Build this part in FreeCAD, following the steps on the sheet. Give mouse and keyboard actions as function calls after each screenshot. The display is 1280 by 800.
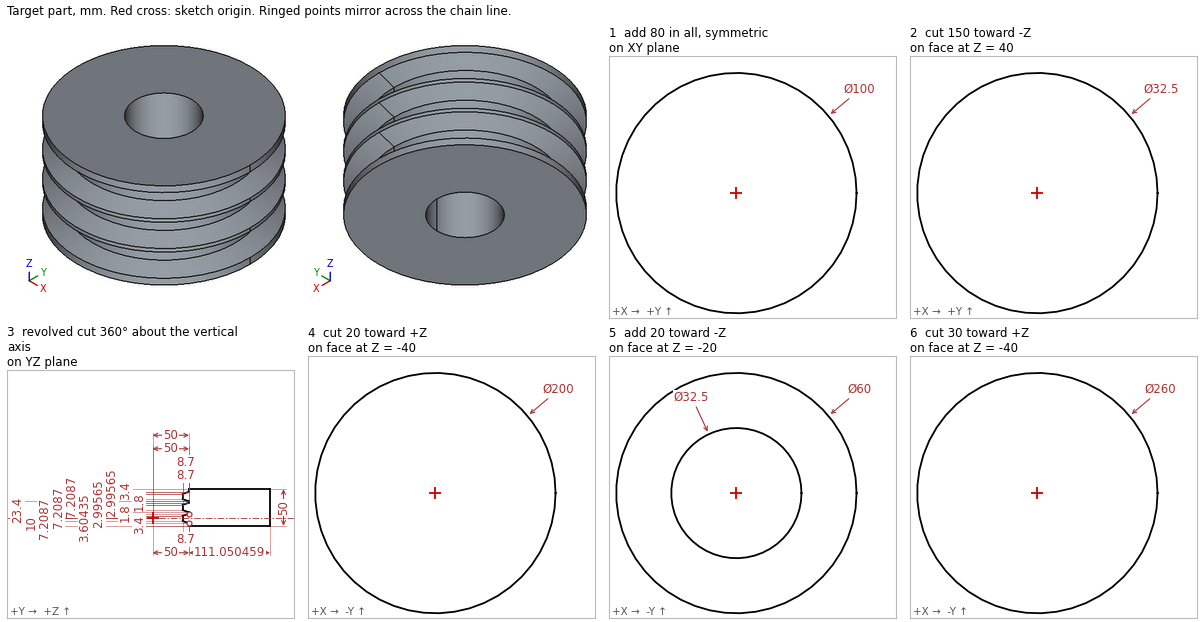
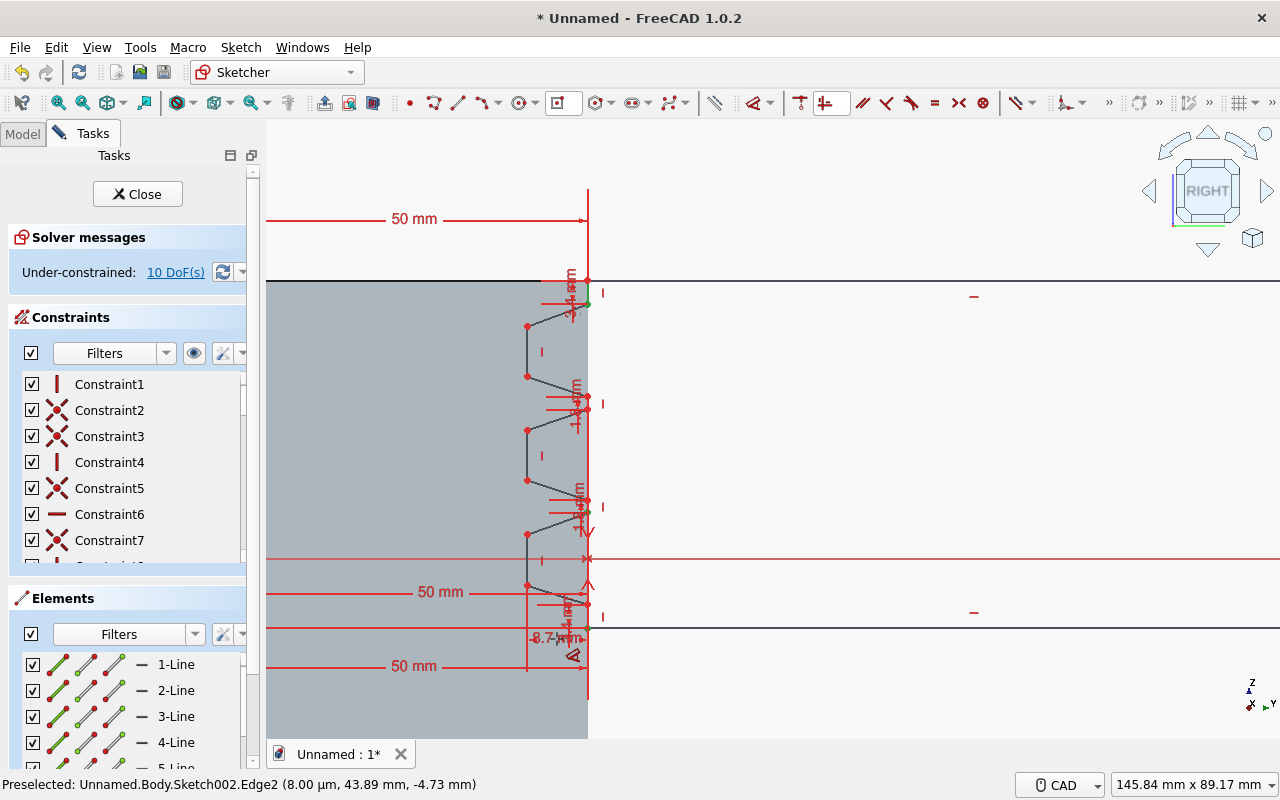
click(570, 311)
click(557, 270)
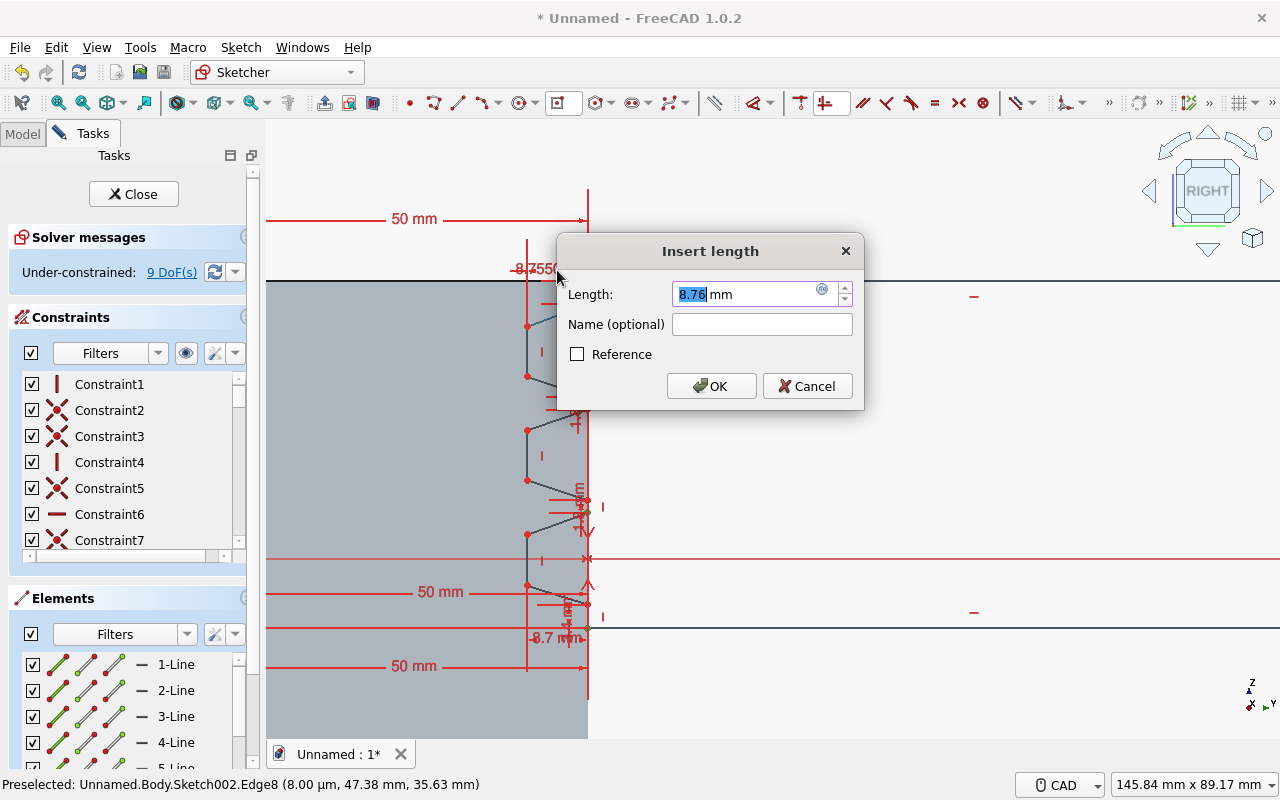
text(8.7)
key(Return)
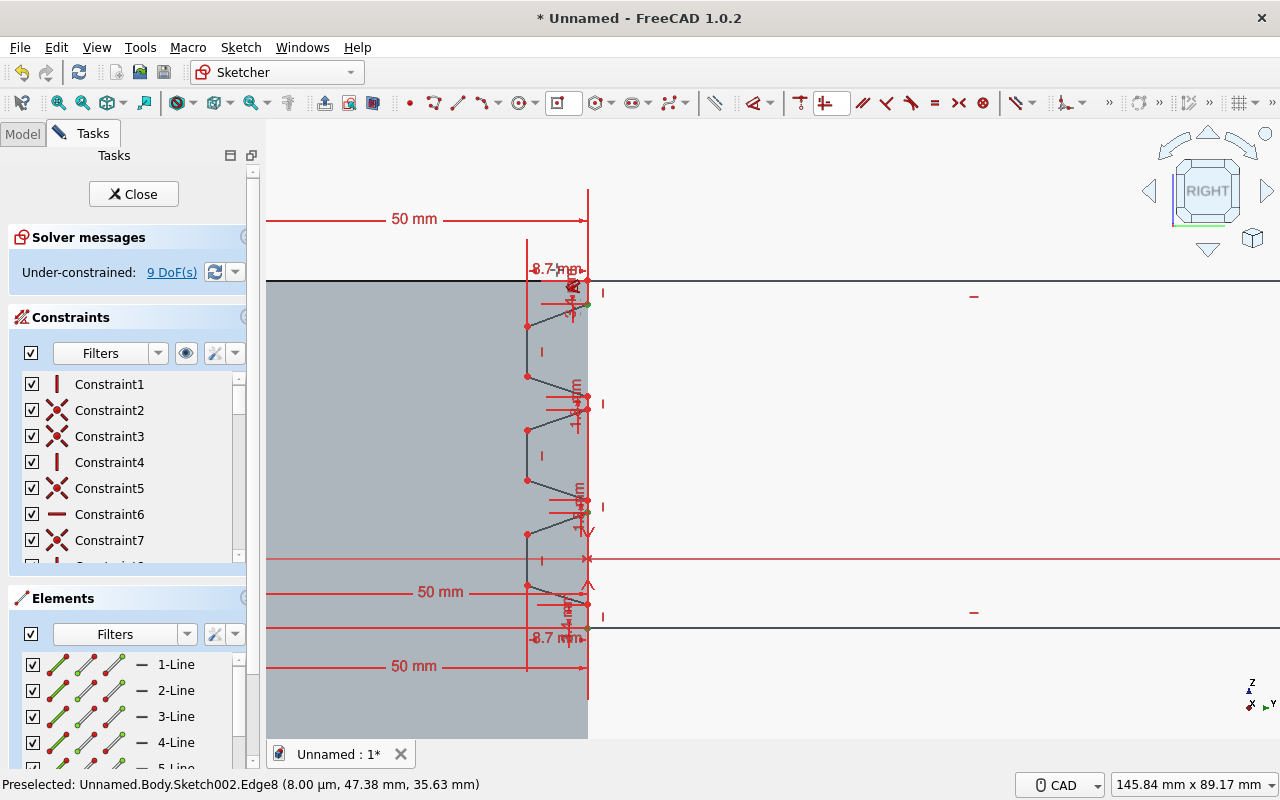
click(570, 416)
click(572, 376)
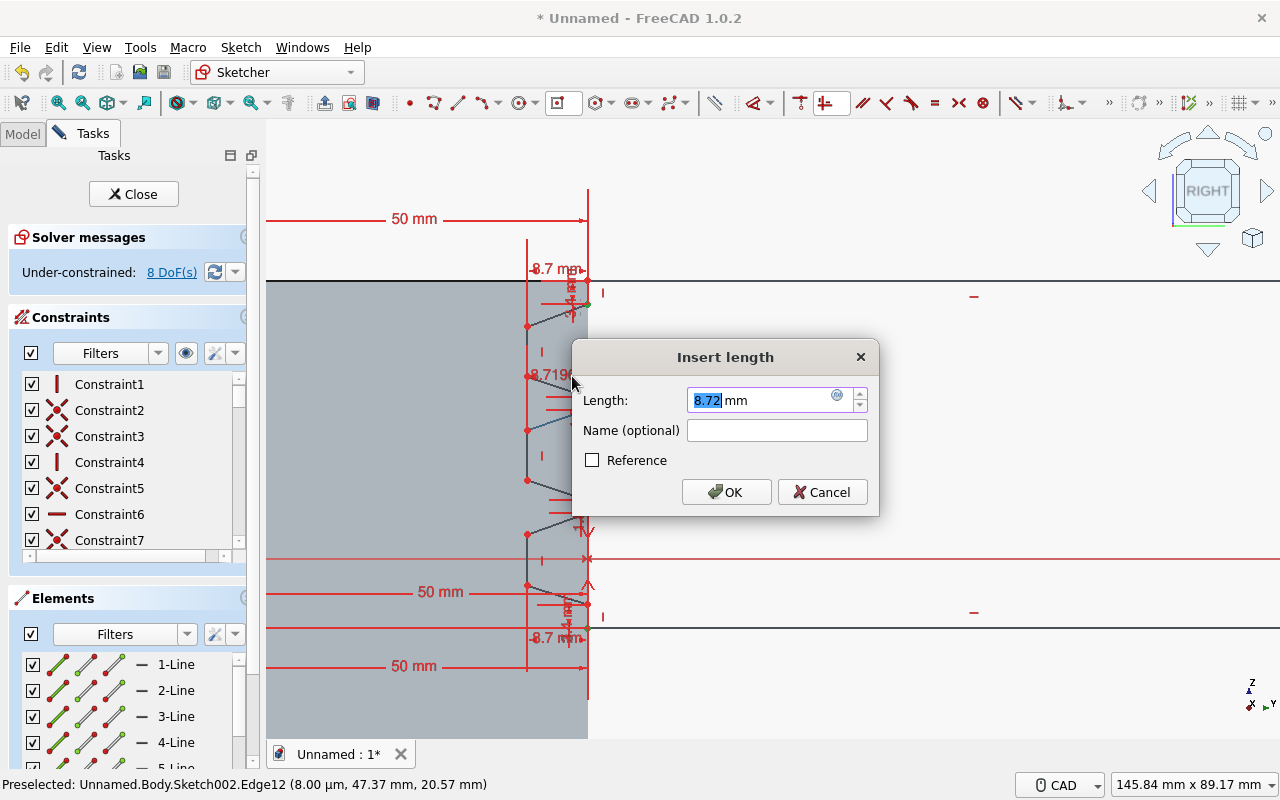
text(8.7)
key(Return)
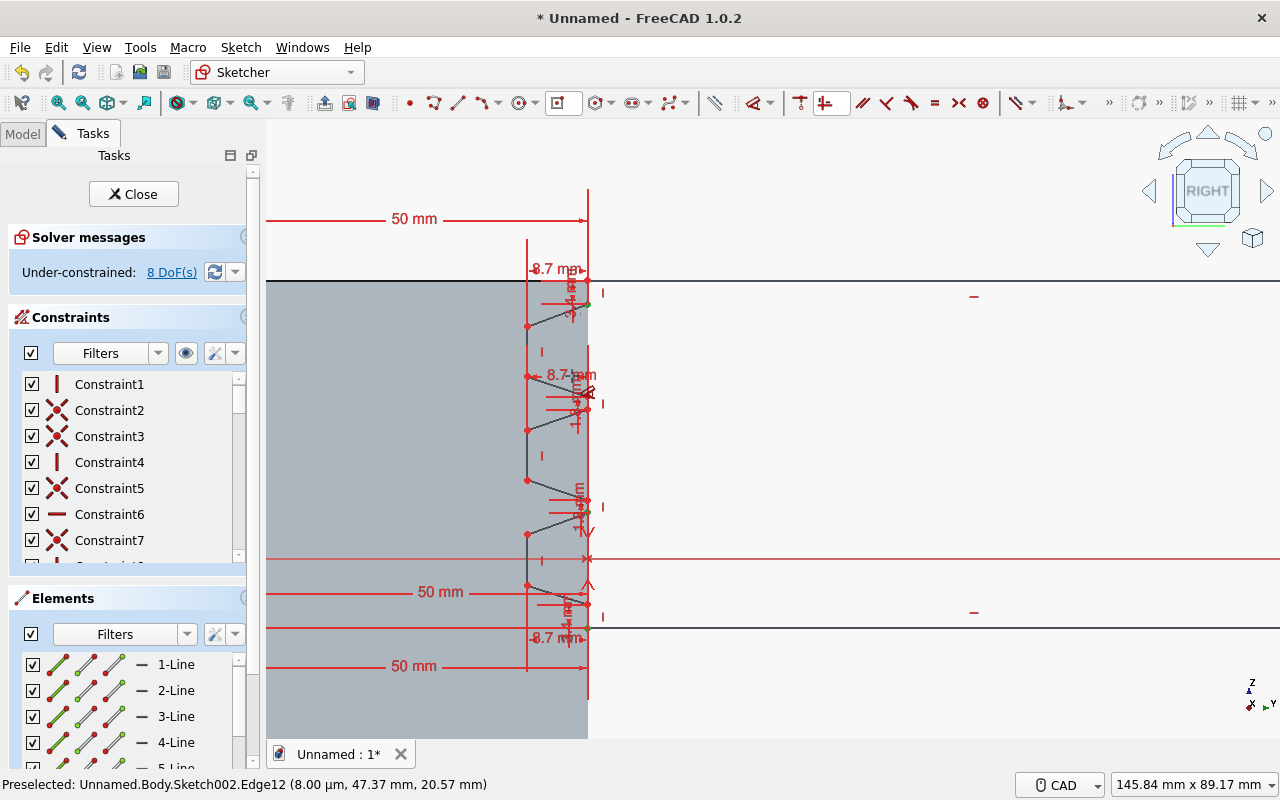
click(588, 397)
click(622, 478)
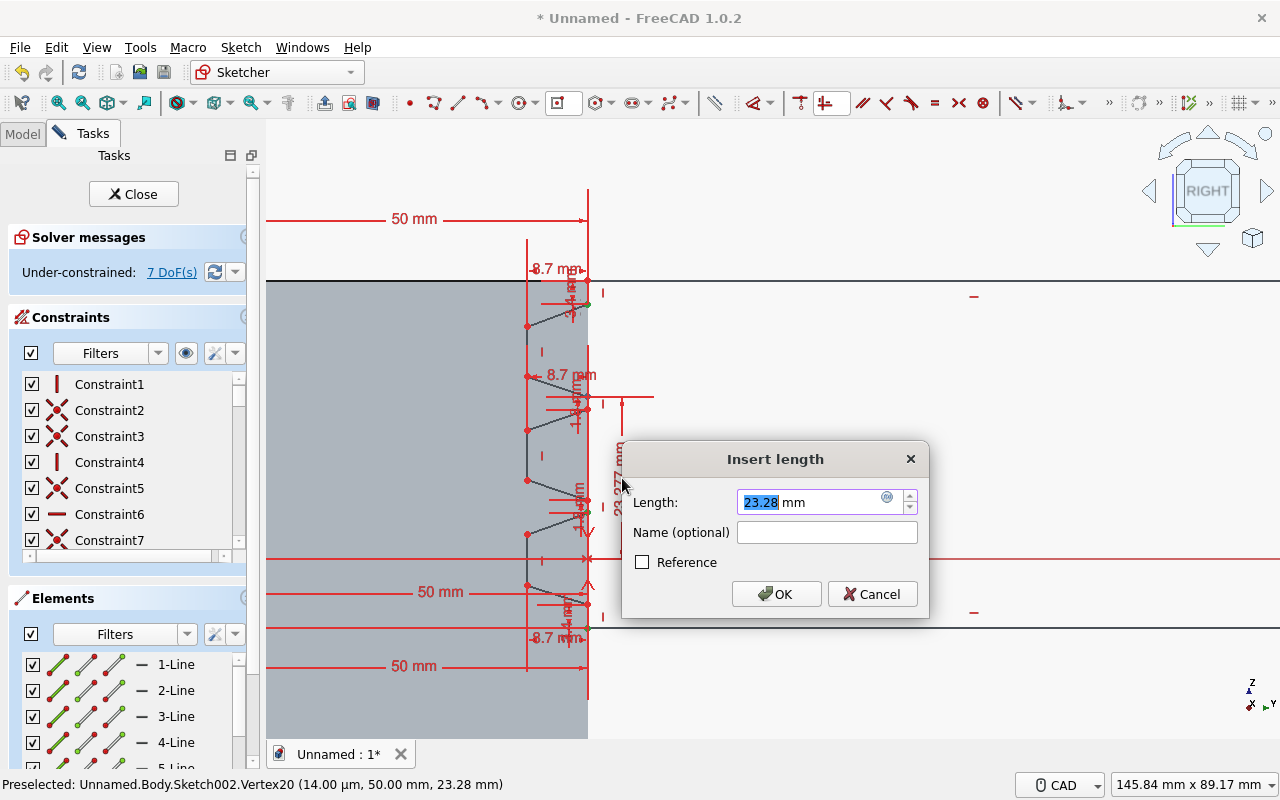
text(23.4)
key(Return)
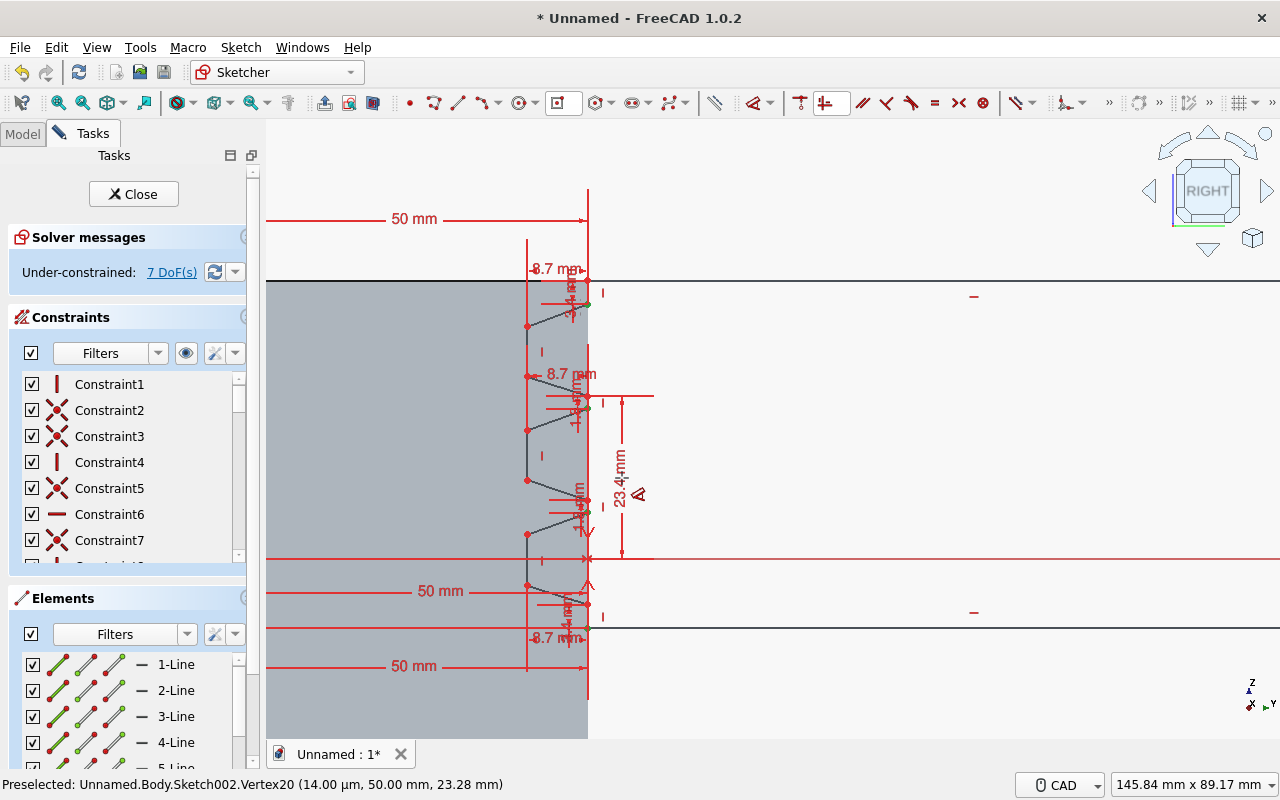
click(527, 571)
click(493, 572)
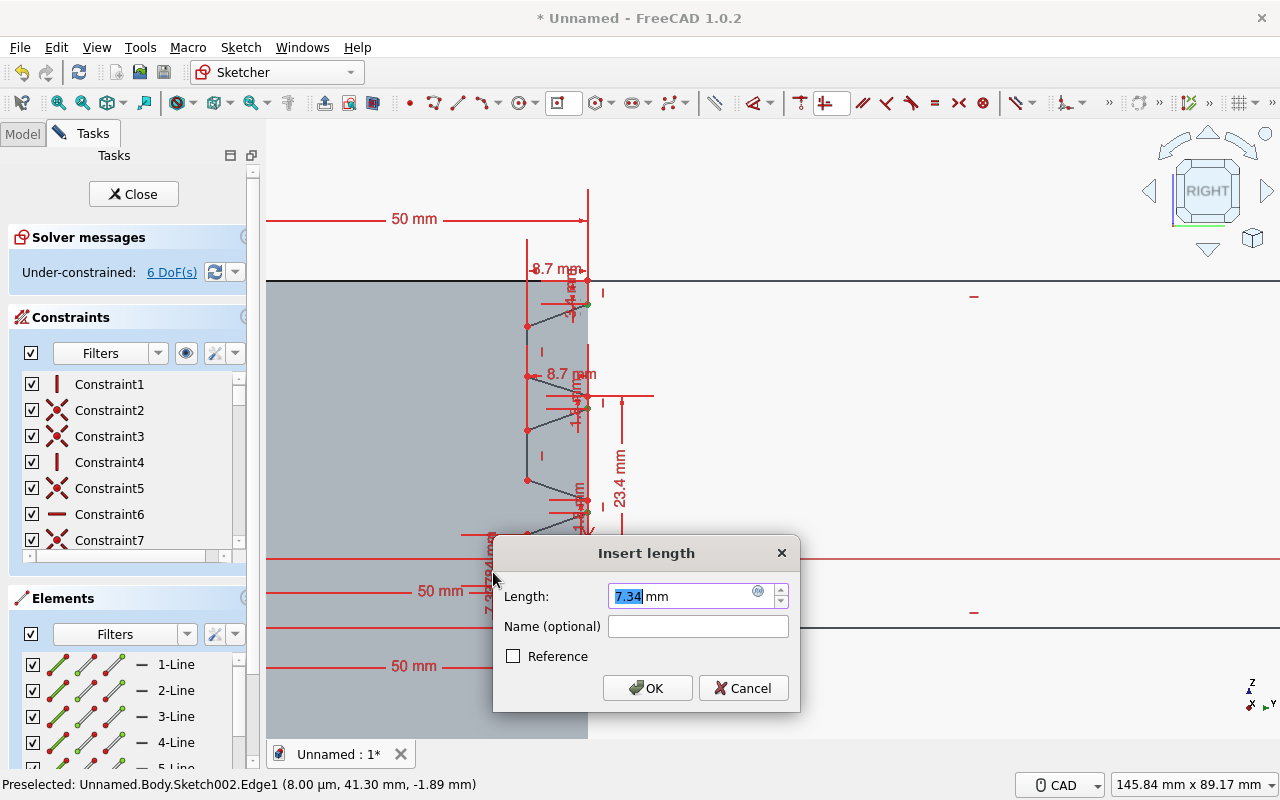
text(7.2087)
key(Return)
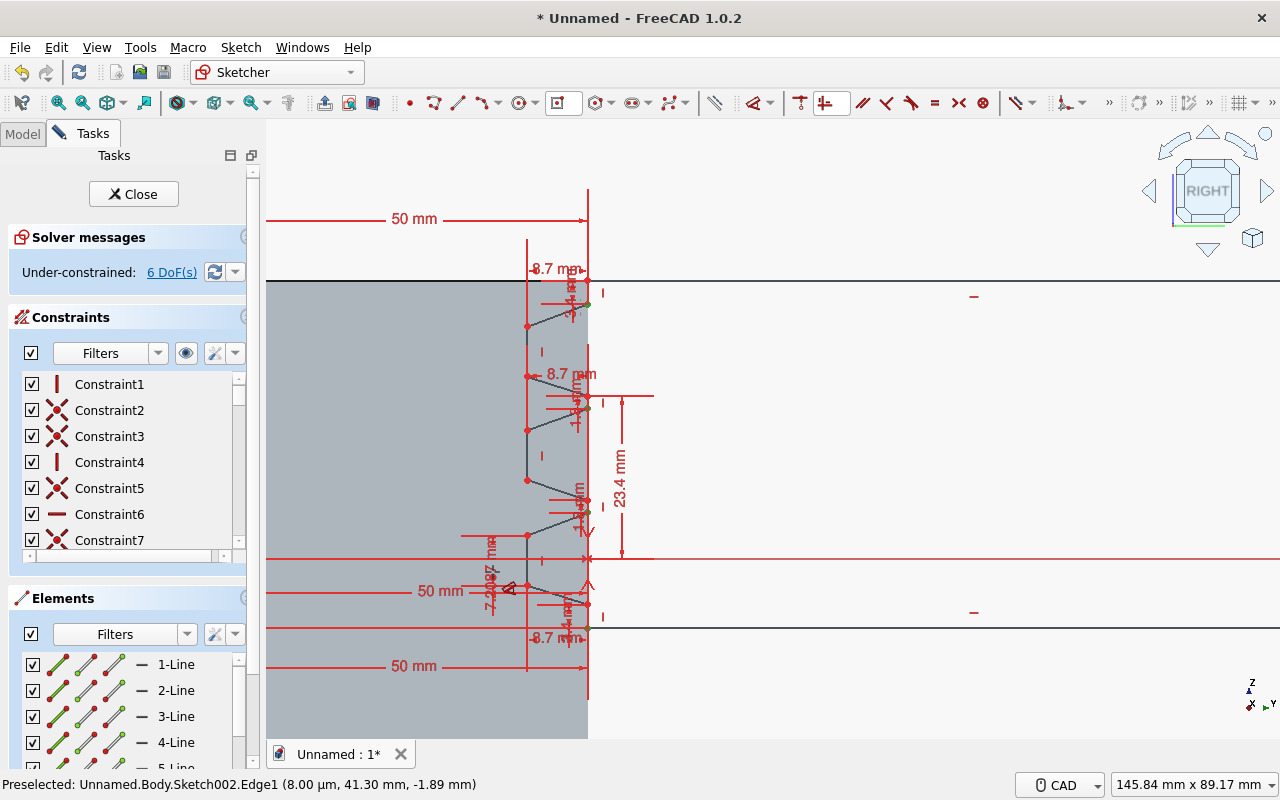
click(527, 342)
click(493, 352)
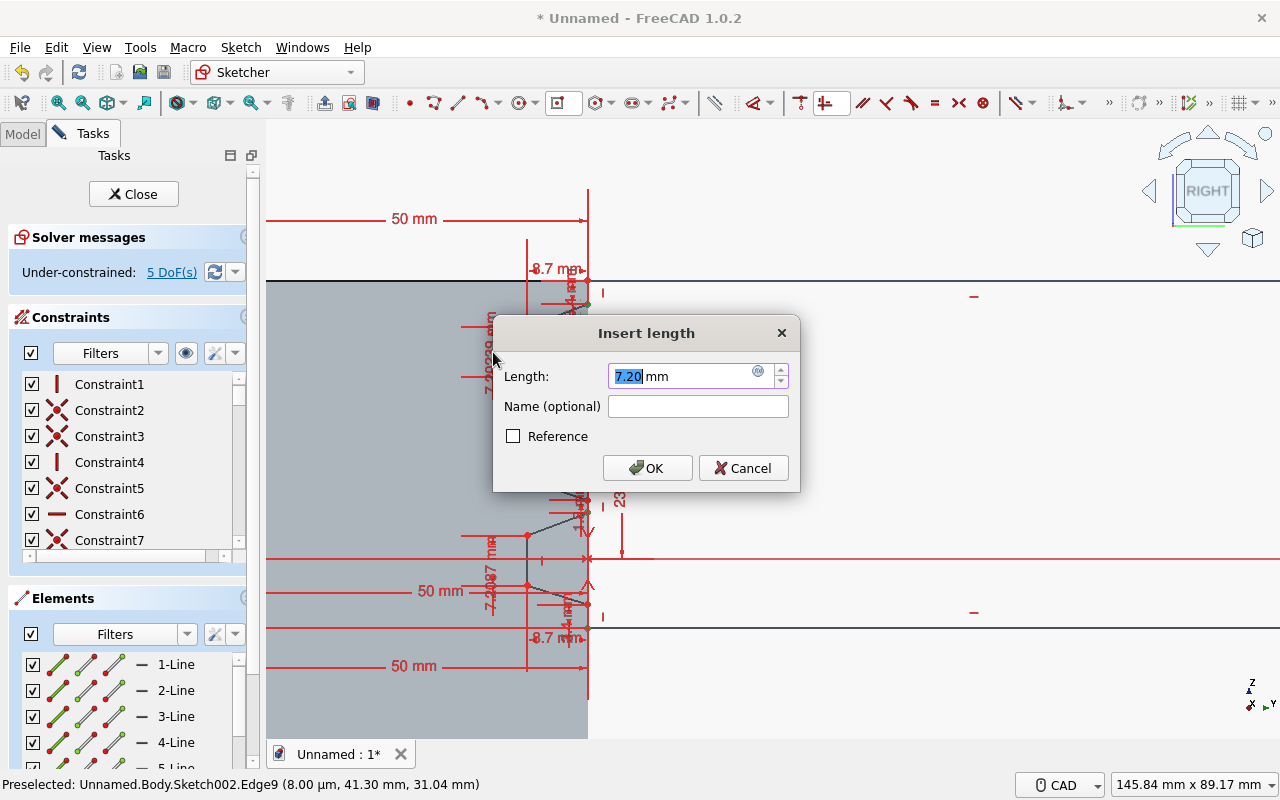
text(7.2087)
key(Return)